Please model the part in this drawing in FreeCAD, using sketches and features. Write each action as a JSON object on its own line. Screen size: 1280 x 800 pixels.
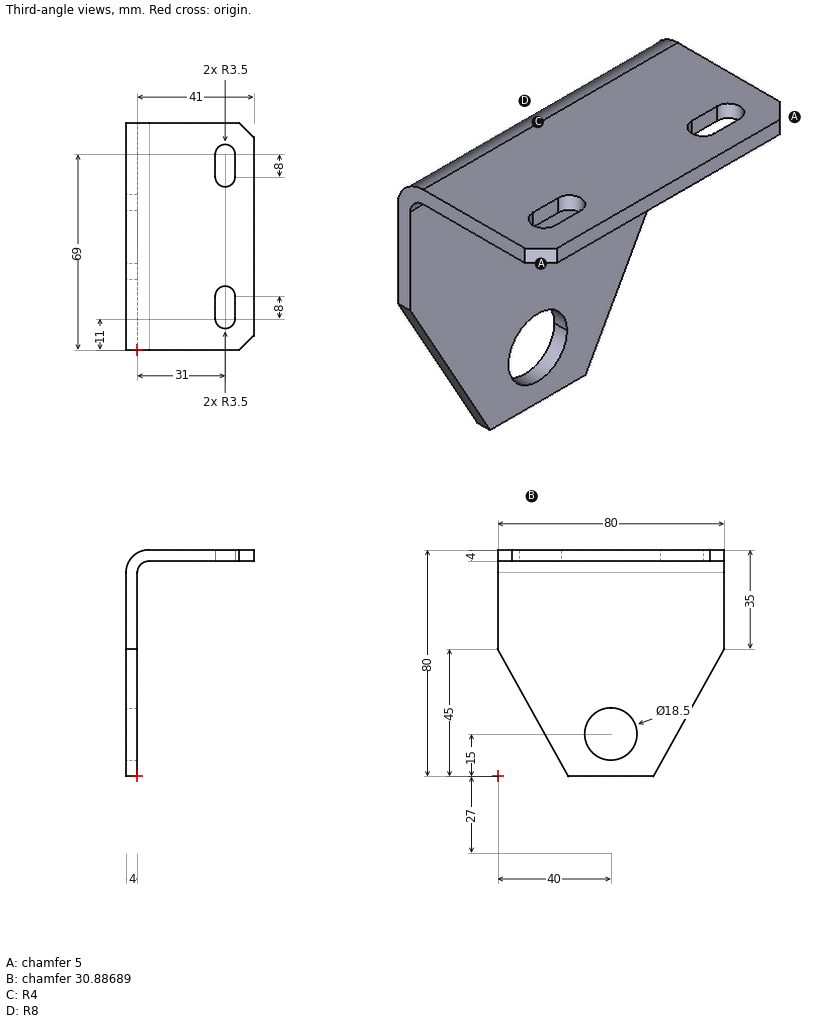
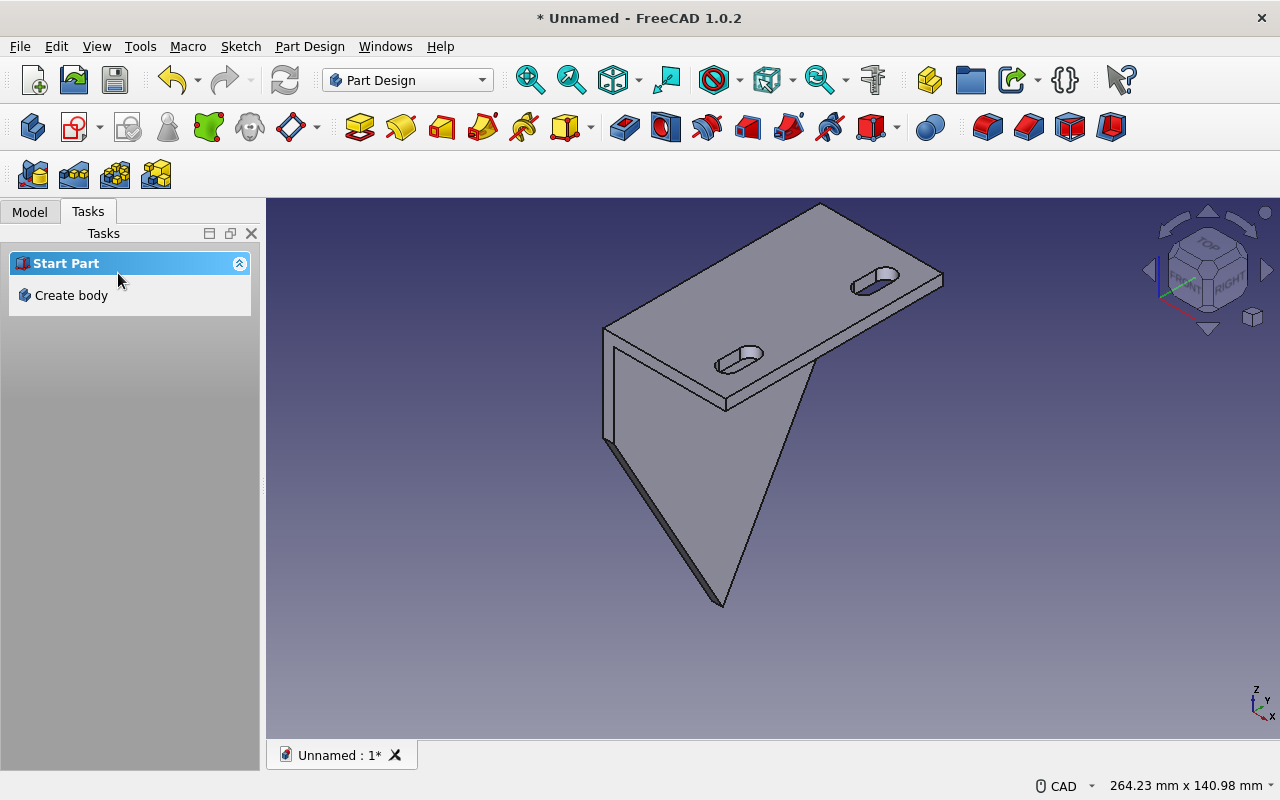
{"action": "left_click", "coordinate": [723, 445]}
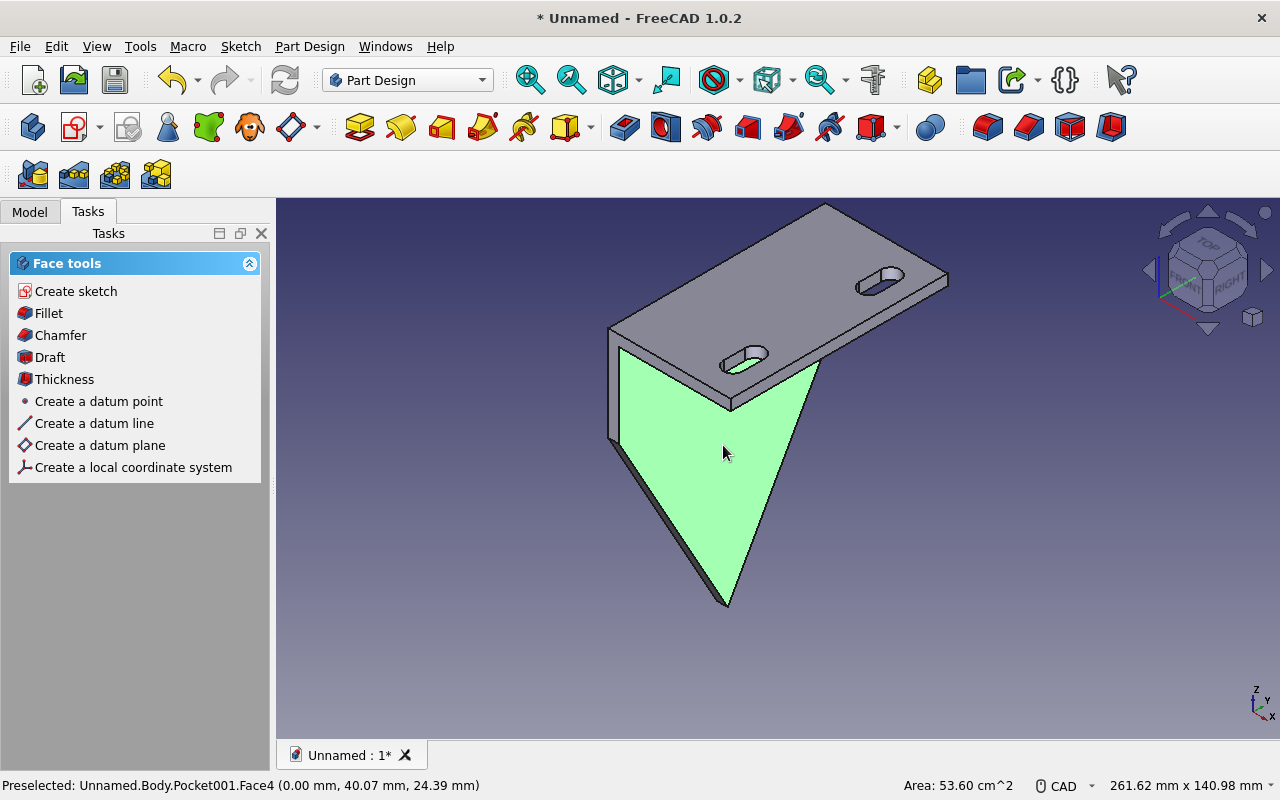
{"action": "left_click", "coordinate": [74, 128]}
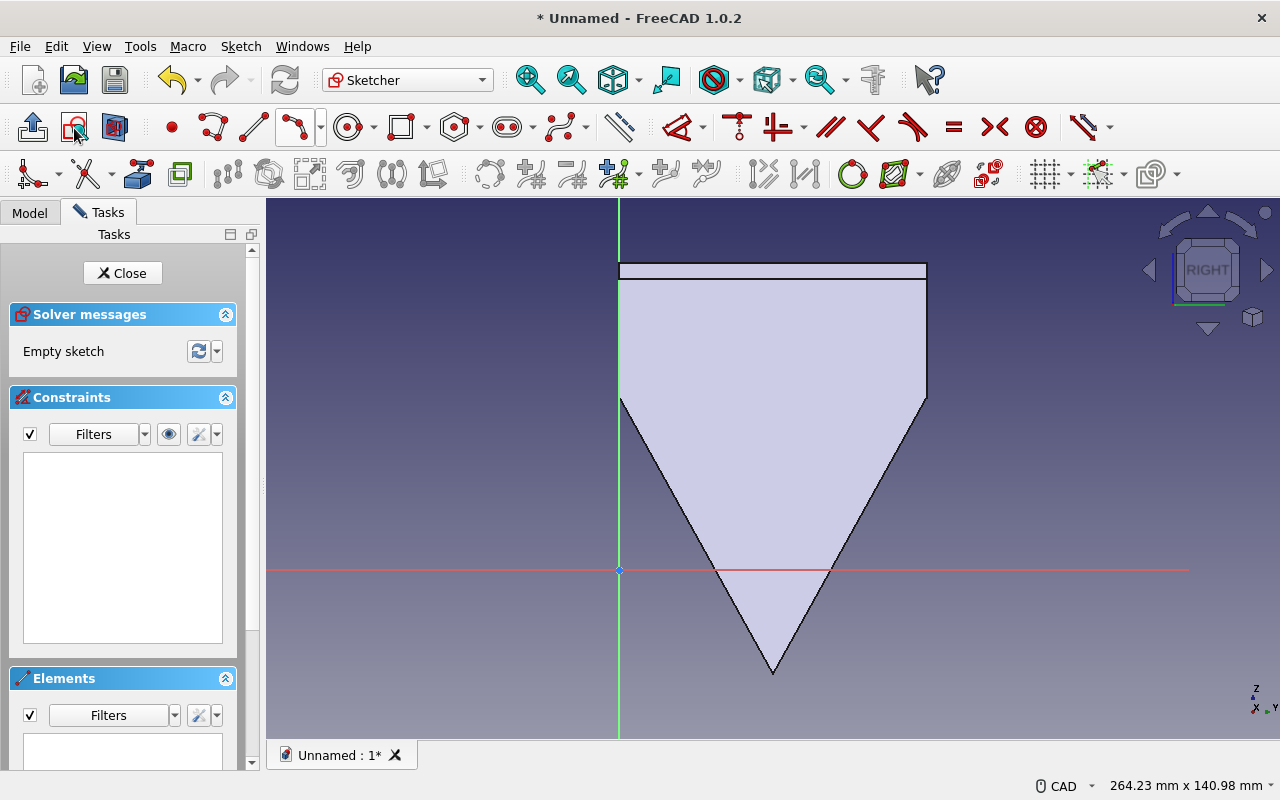
{"action": "scroll", "coordinate": [790, 524], "scroll_direction": "up", "scroll_amount": 8}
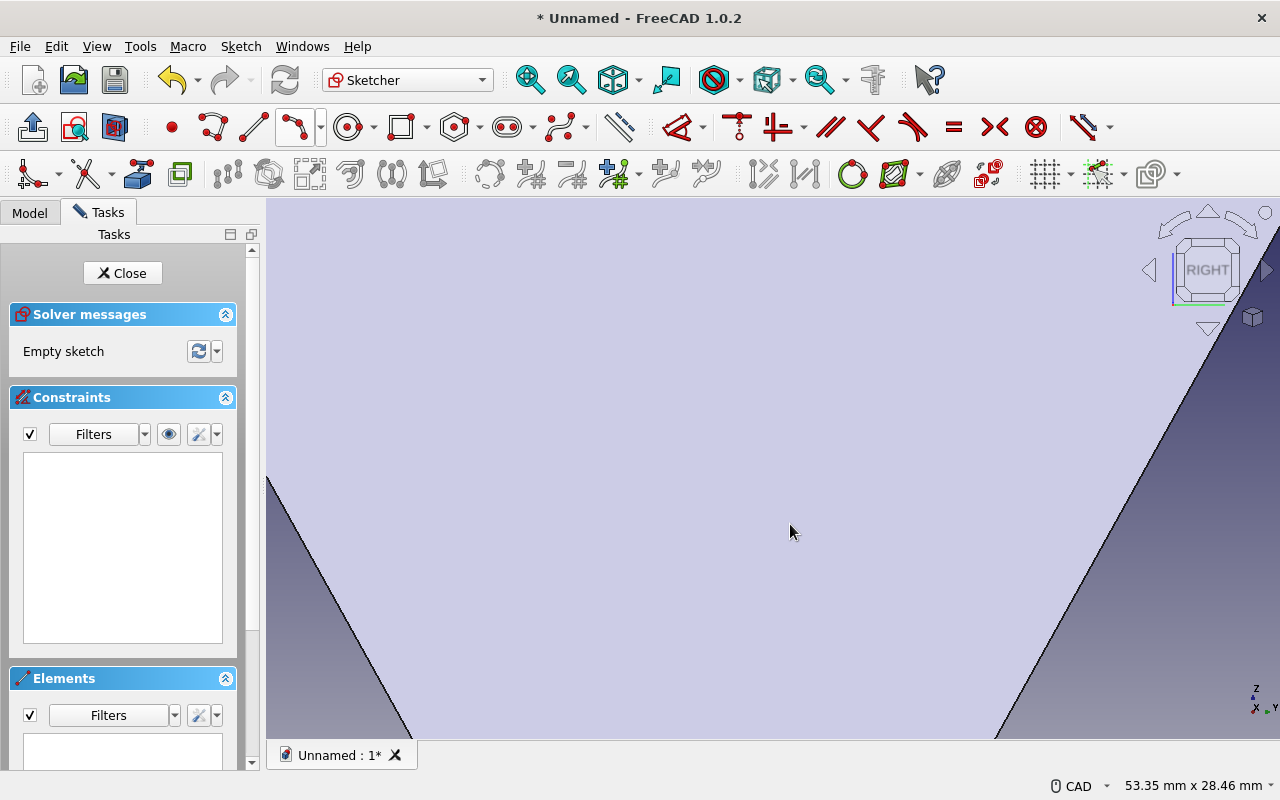
{"action": "key", "text": "g c"}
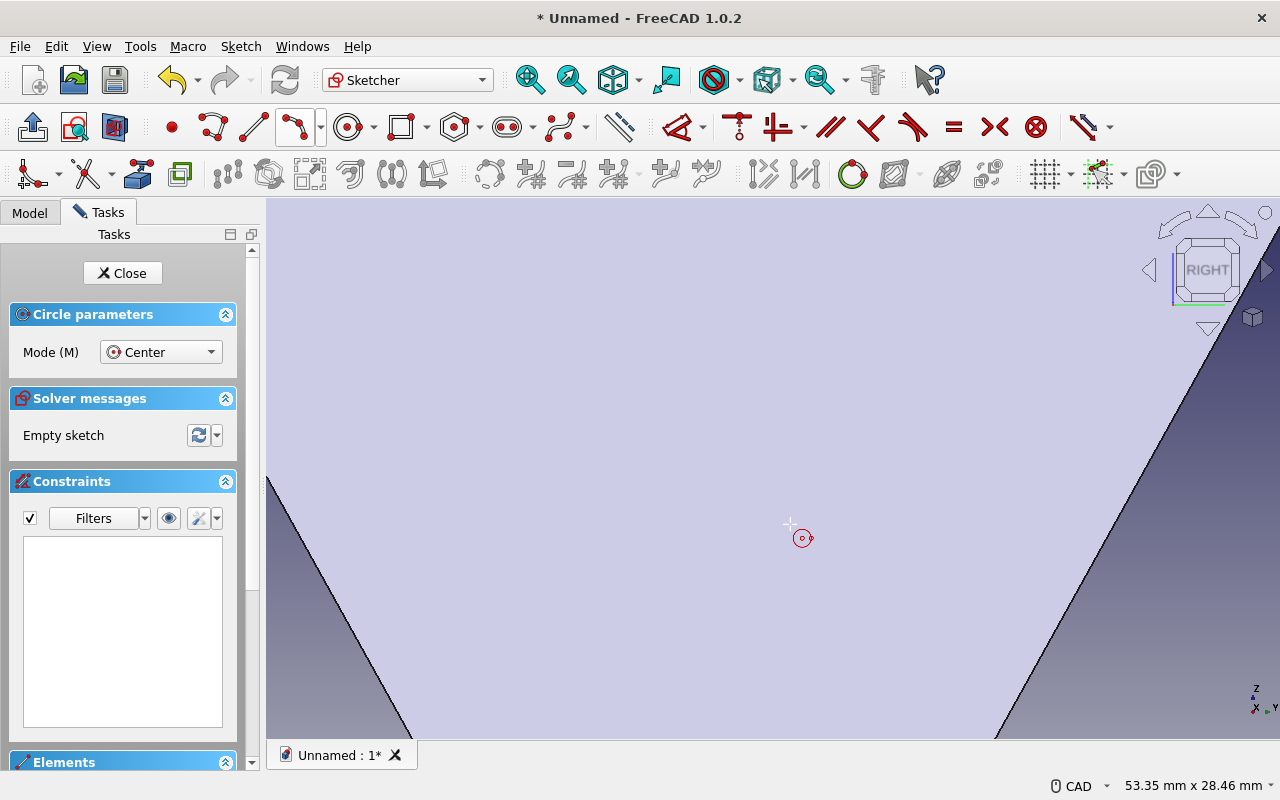
{"action": "left_click", "coordinate": [704, 465]}
{"action": "left_click", "coordinate": [828, 341]}
{"action": "key", "text": "Escape"}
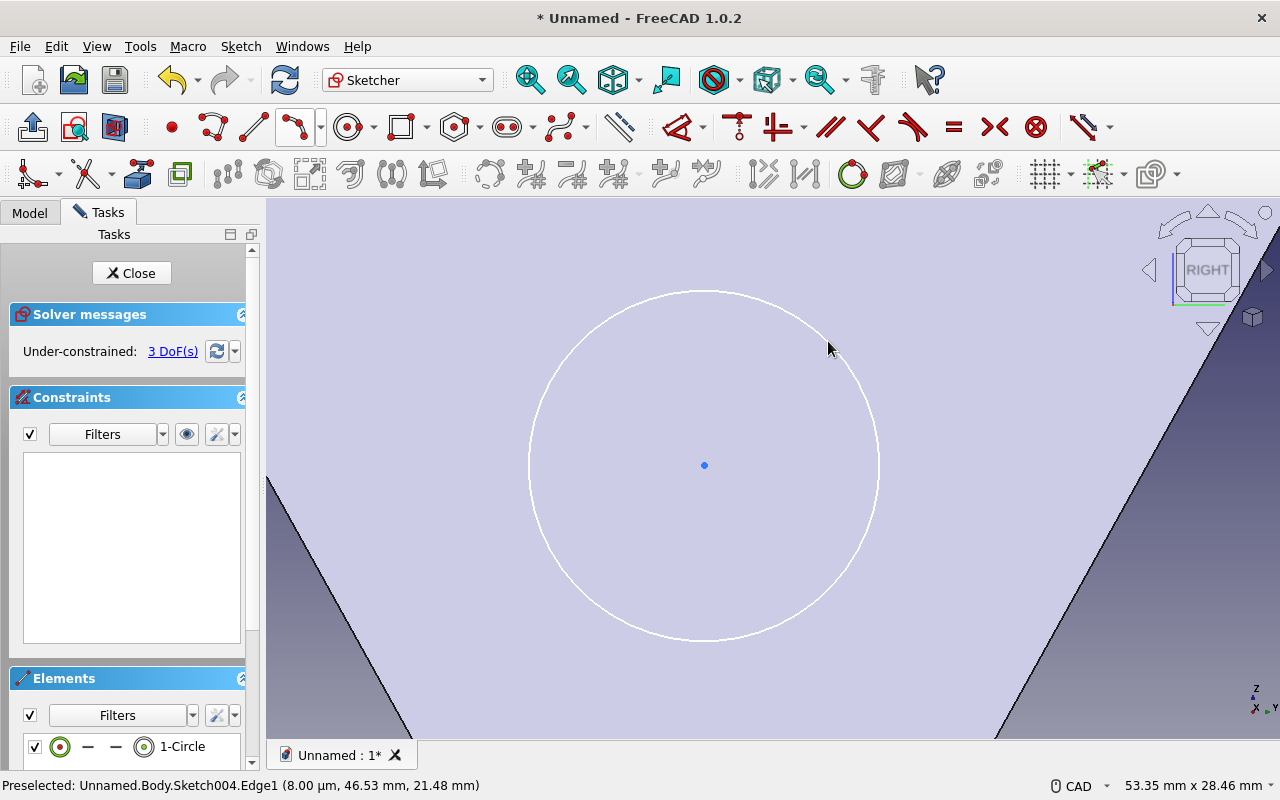
{"action": "key", "text": "d"}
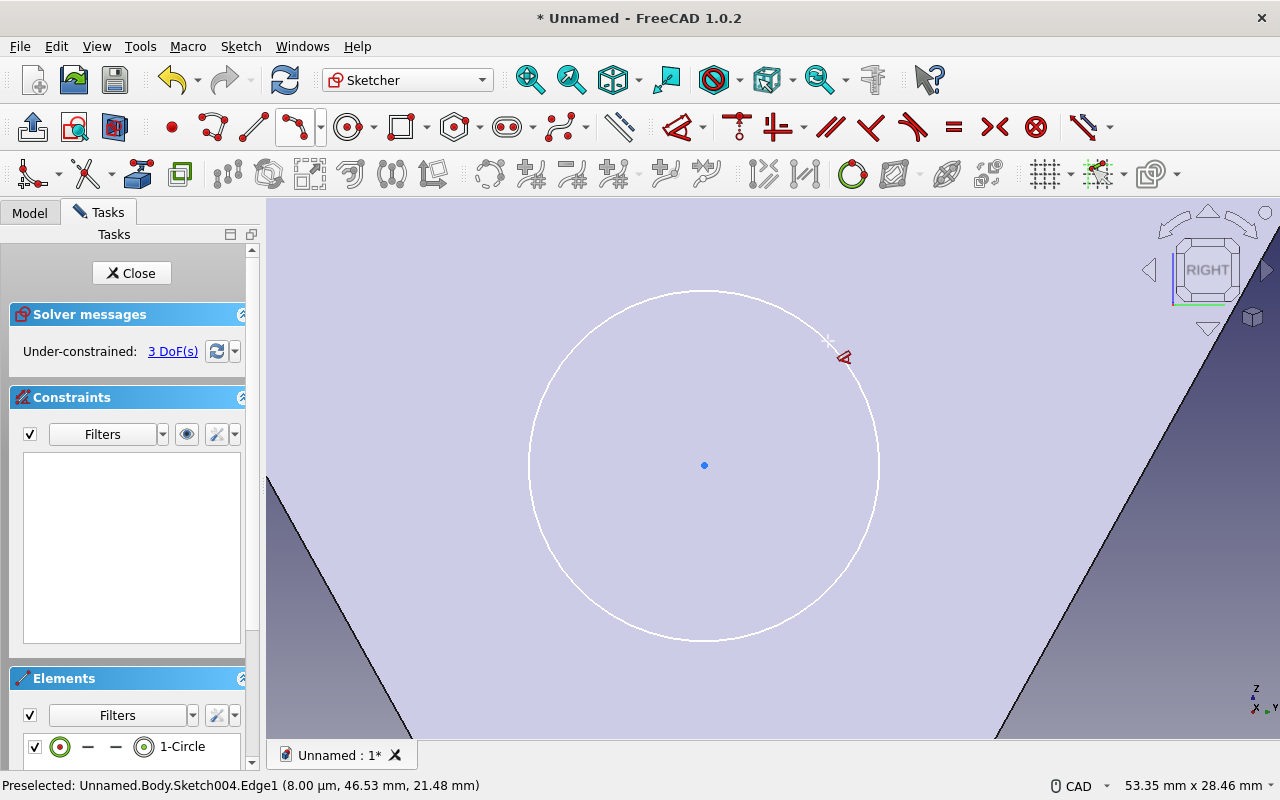
{"action": "left_click", "coordinate": [828, 342]}
{"action": "left_click", "coordinate": [851, 319]}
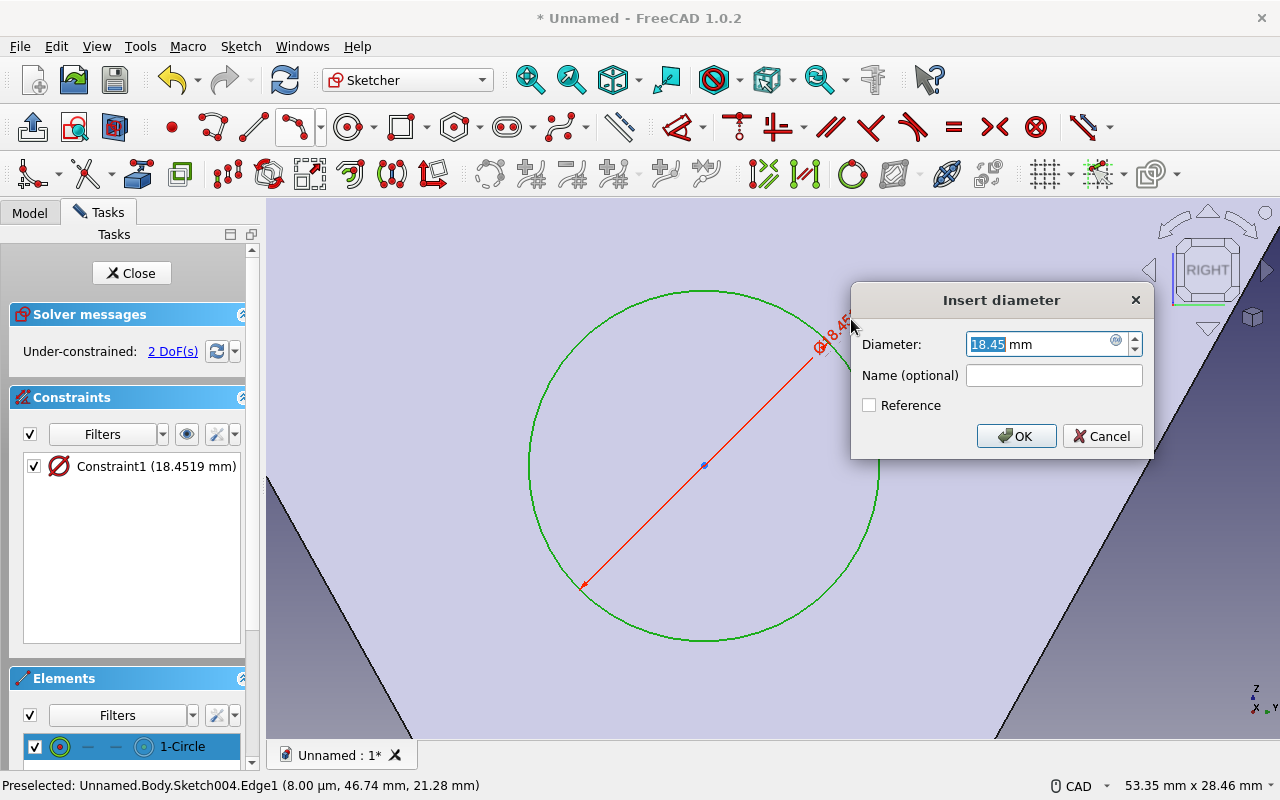
{"action": "type", "text": "18.5"}
{"action": "key", "text": "Return"}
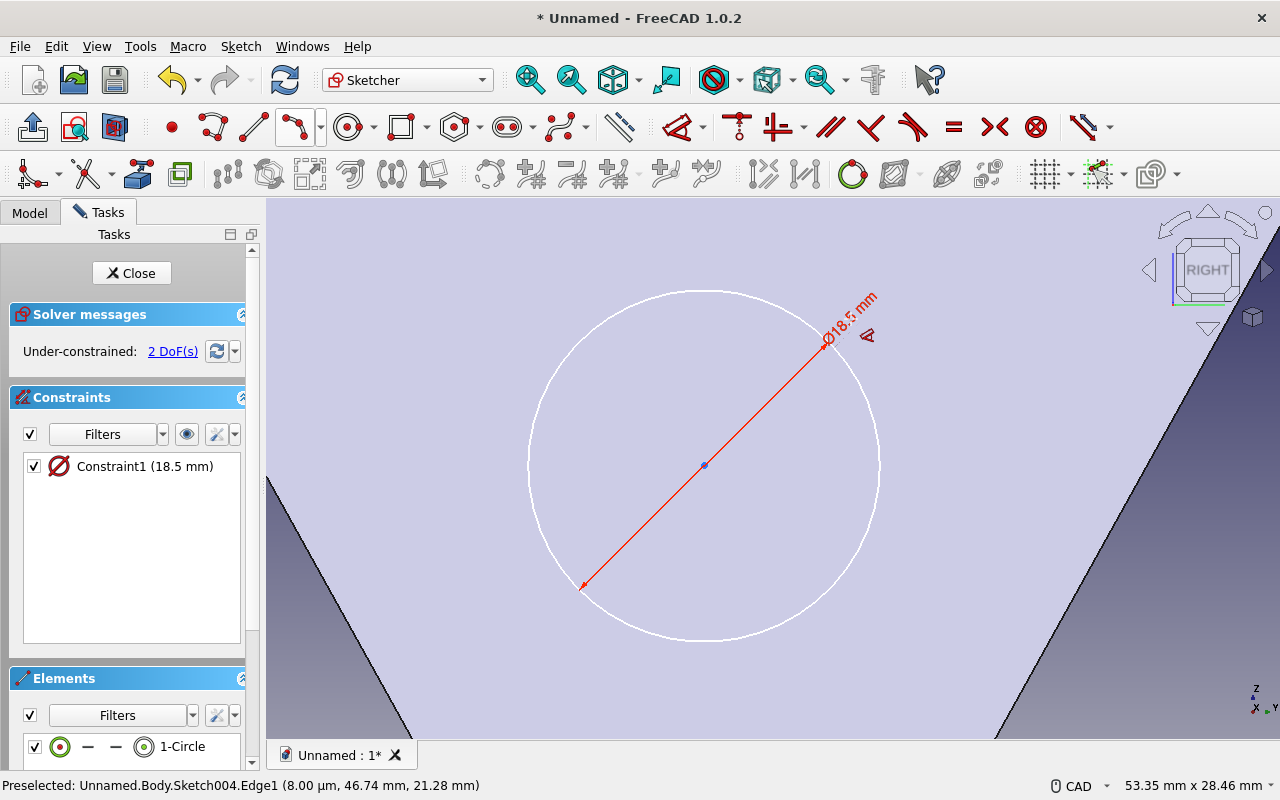
{"action": "left_click", "coordinate": [704, 466]}
{"action": "left_click", "coordinate": [499, 432]}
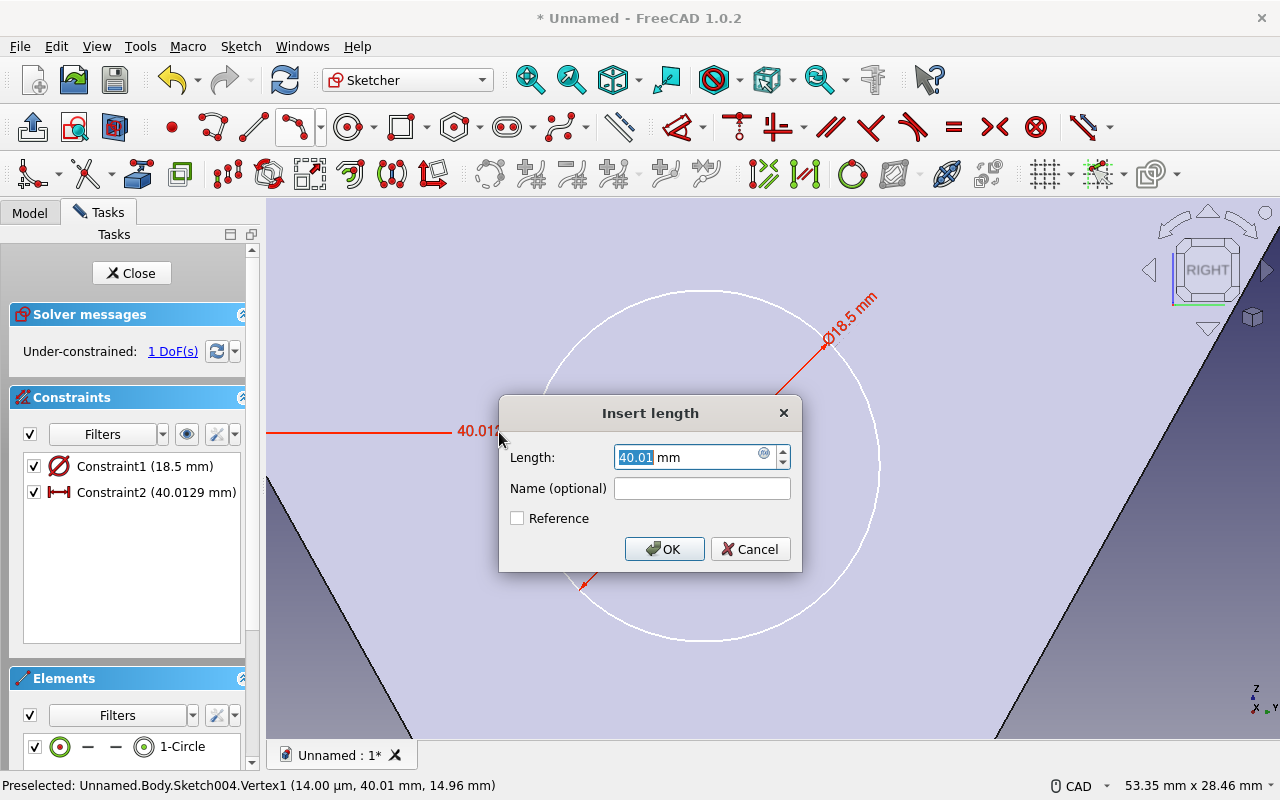
{"action": "type", "text": "40"}
{"action": "key", "text": "Return"}